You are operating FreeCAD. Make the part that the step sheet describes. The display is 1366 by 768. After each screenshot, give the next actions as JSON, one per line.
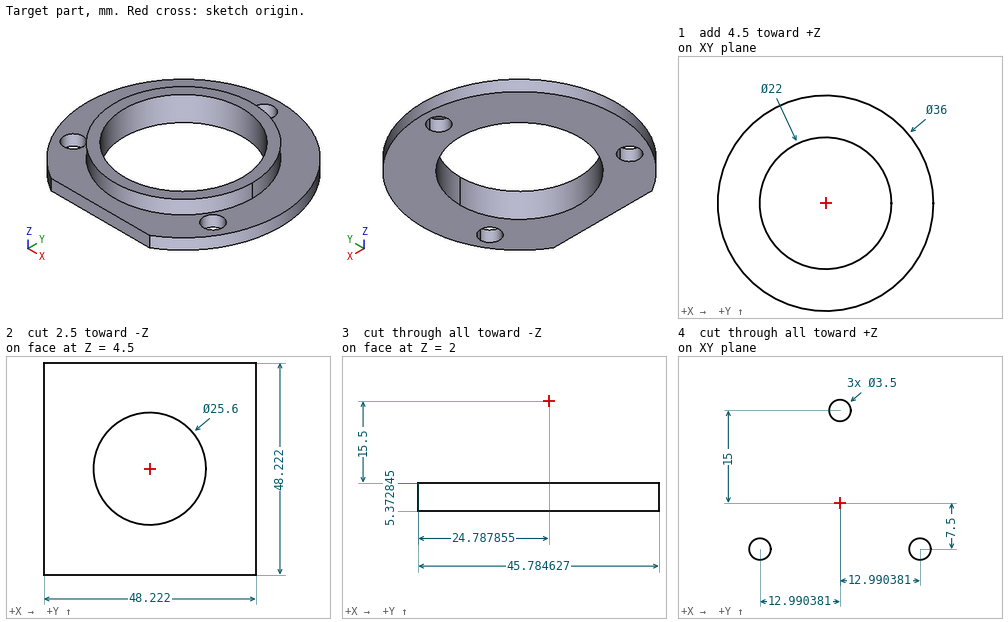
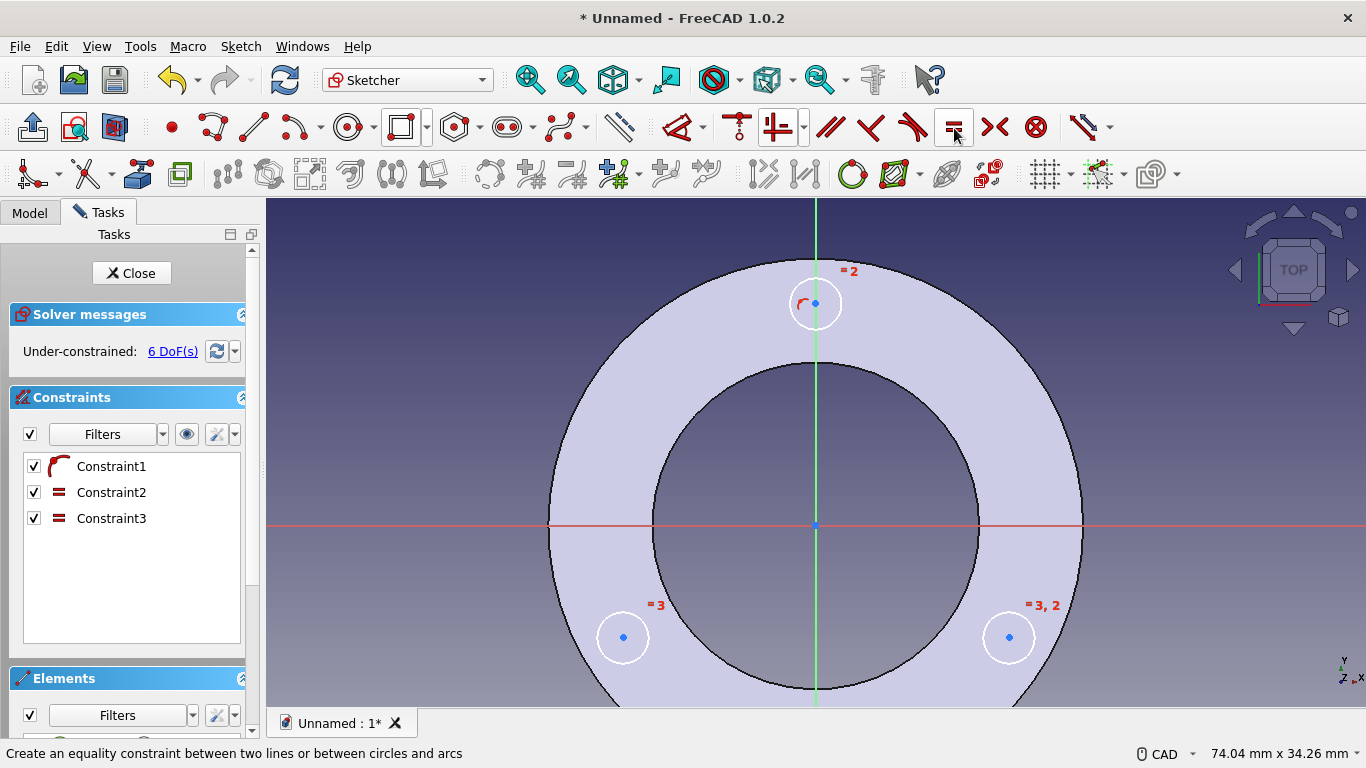
{"action": "left_click", "coordinate": [1009, 638]}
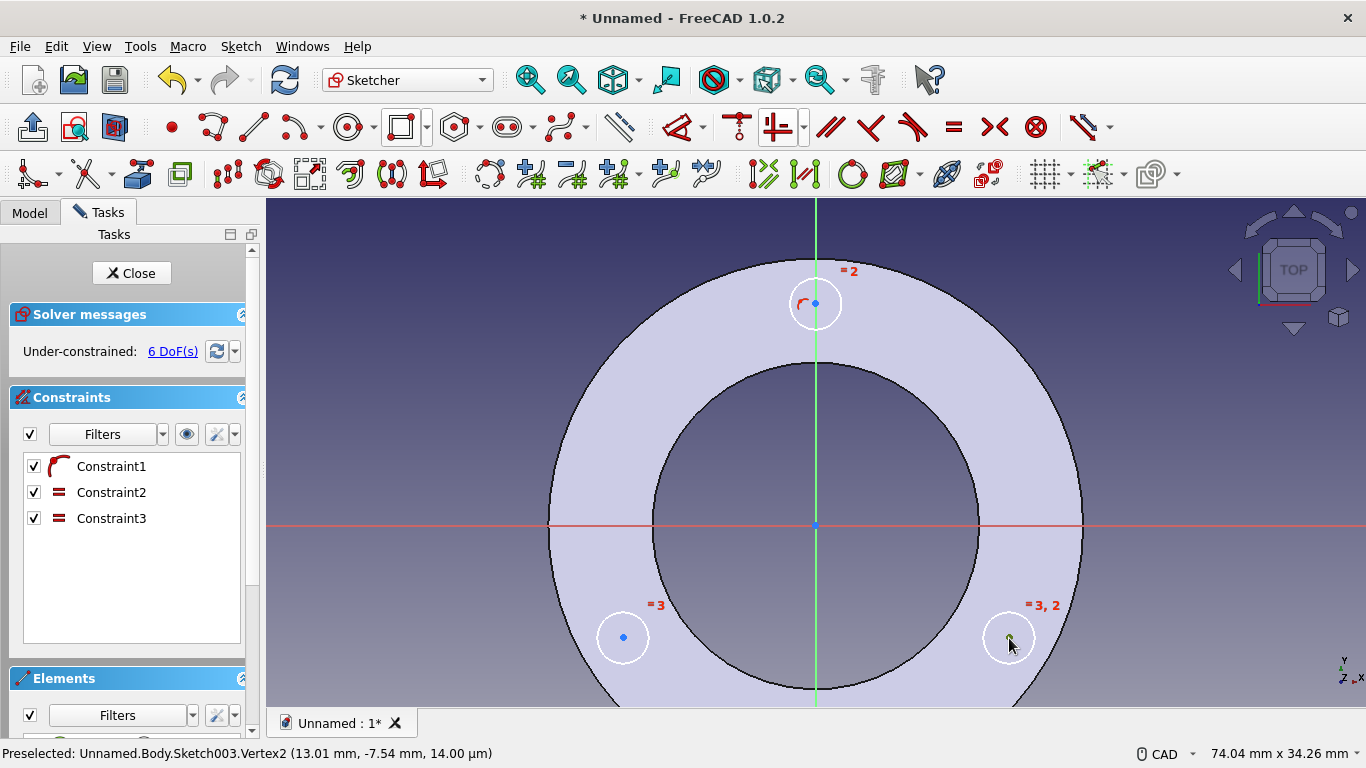
{"action": "left_click", "coordinate": [623, 638]}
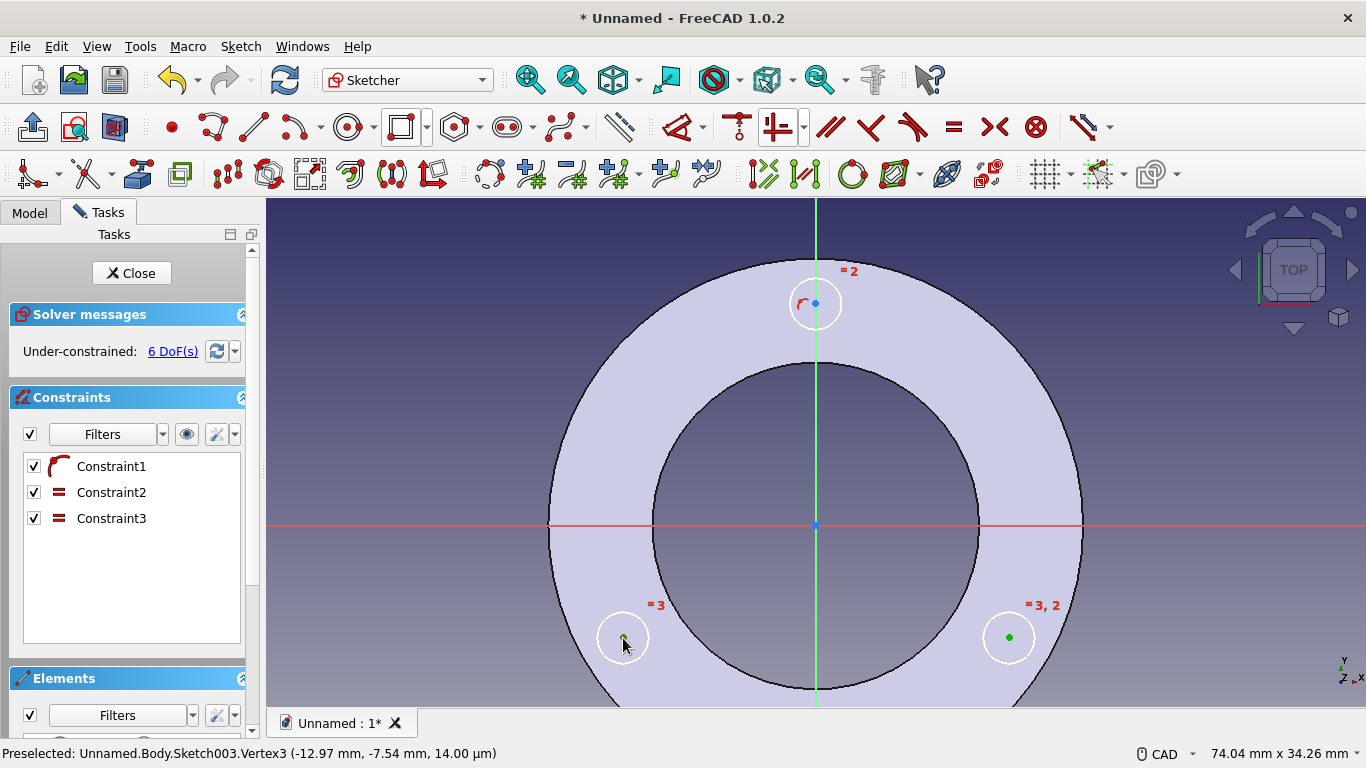
{"action": "left_click", "coordinate": [804, 128]}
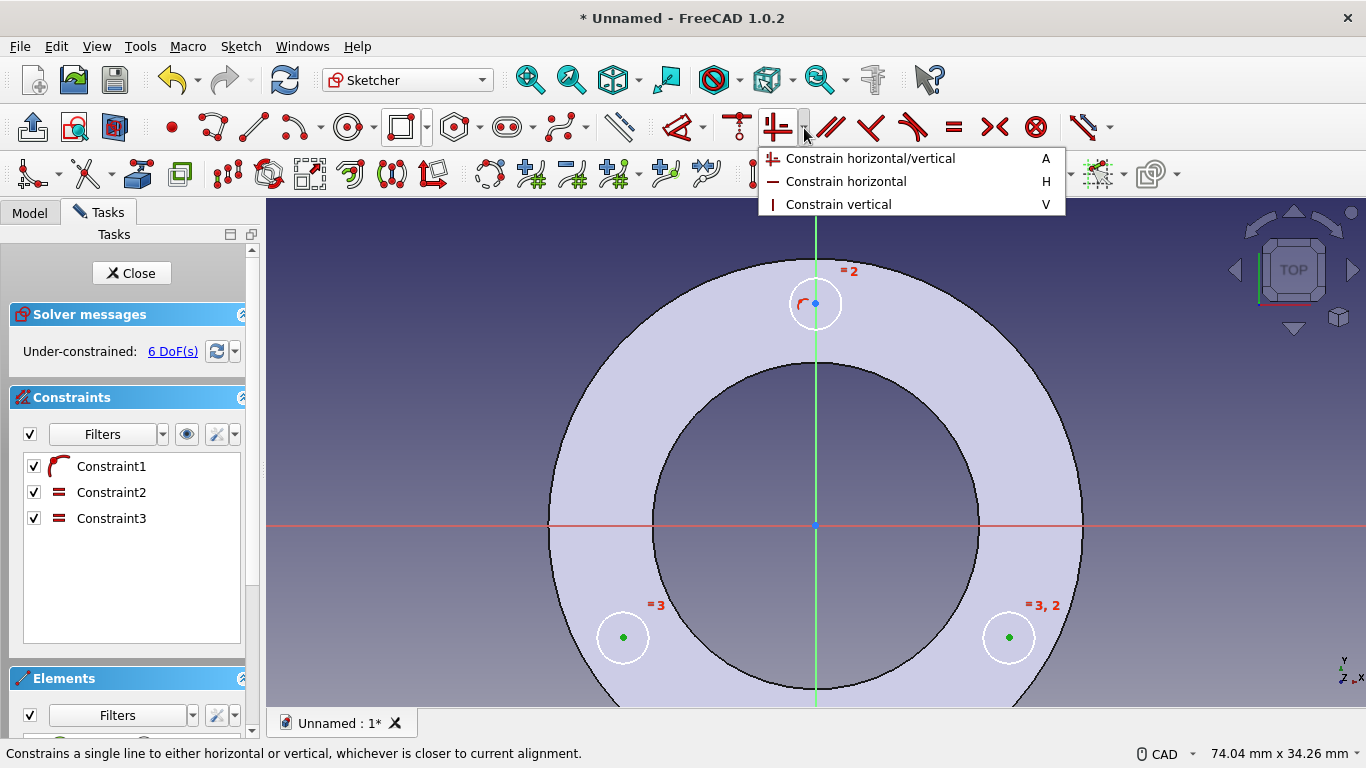
{"action": "left_click", "coordinate": [912, 182]}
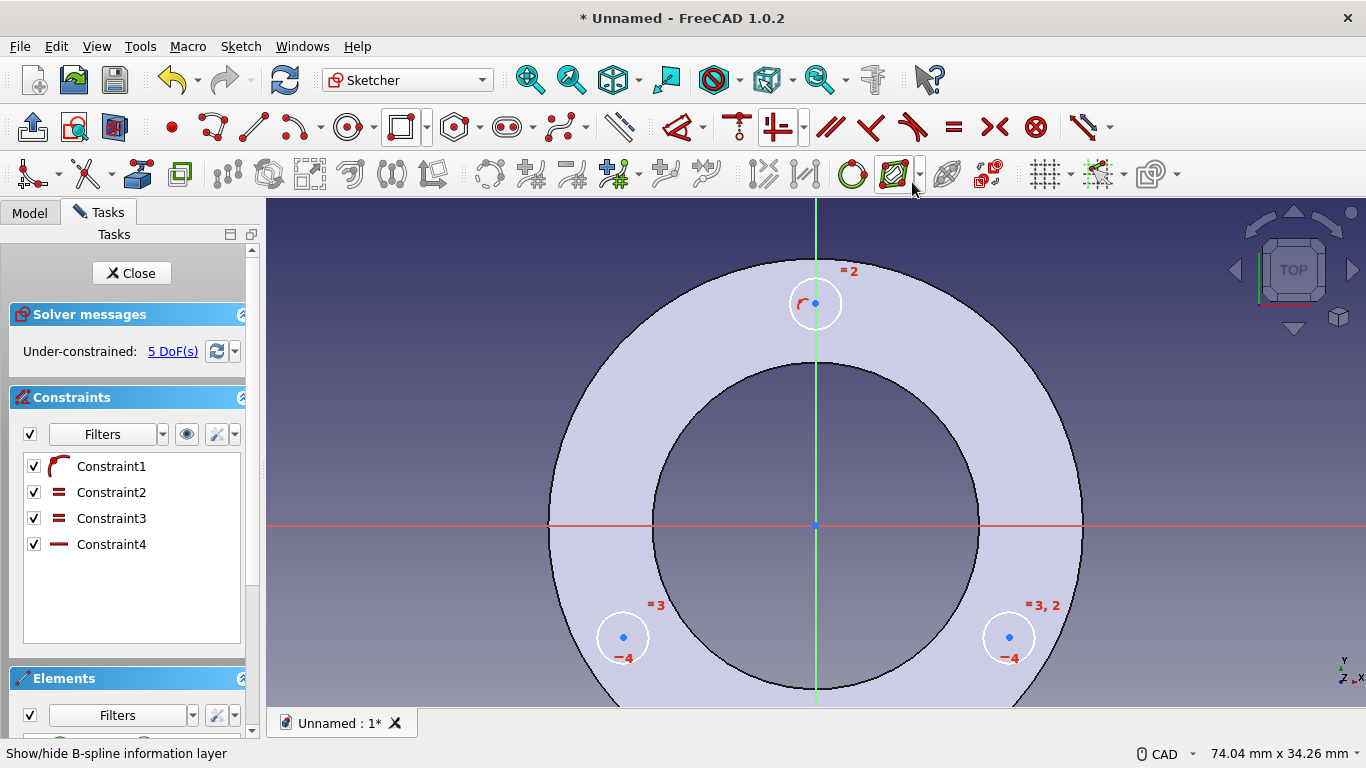
{"action": "left_click", "coordinate": [676, 128]}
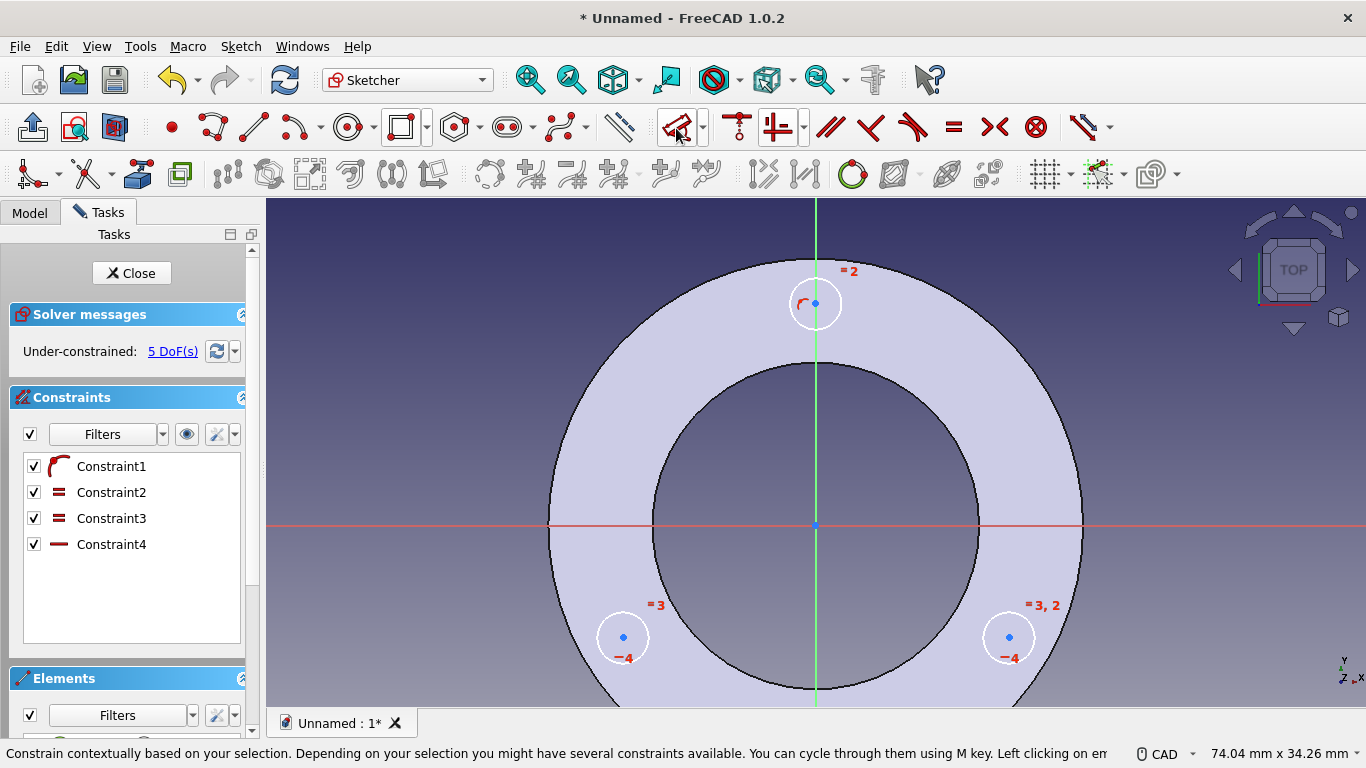
{"action": "left_click", "coordinate": [834, 286]}
{"action": "left_click", "coordinate": [857, 264]}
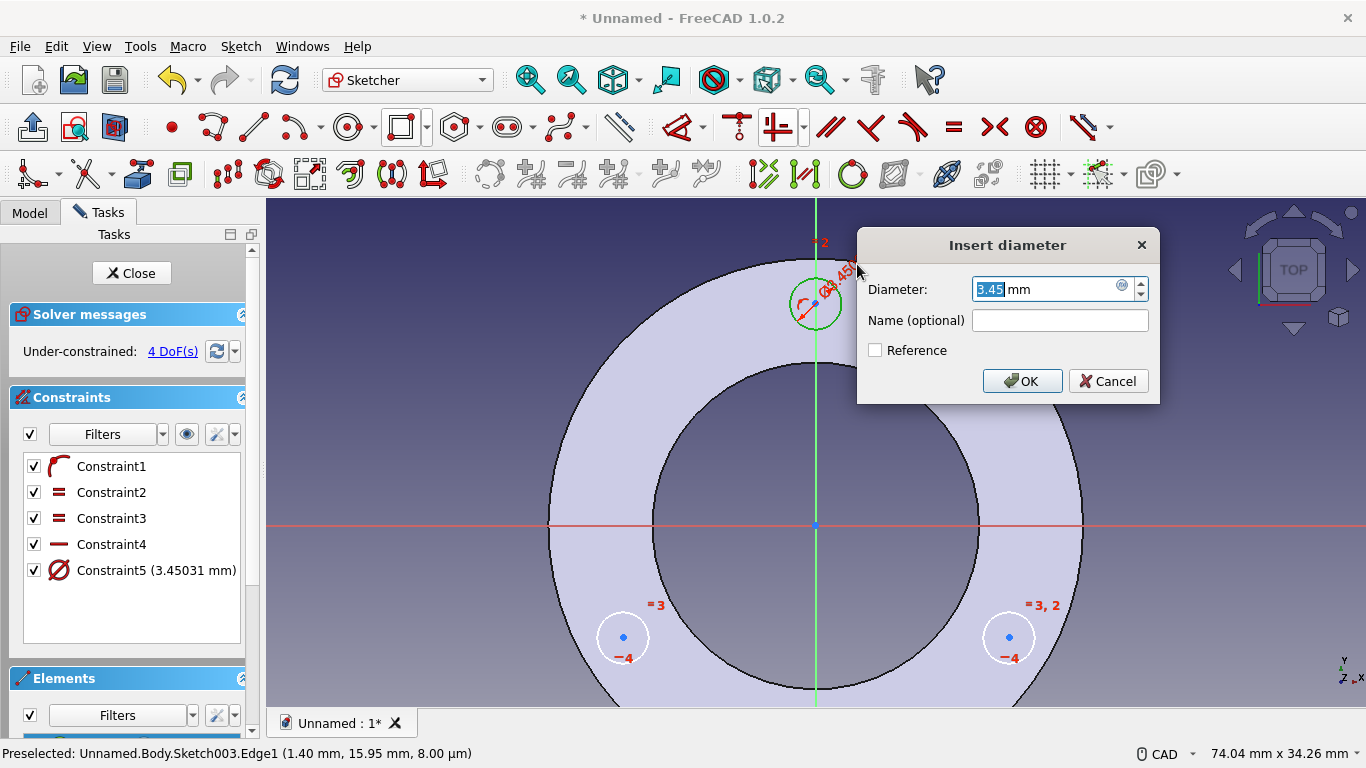
{"action": "type", "text": "3.5"}
{"action": "key", "text": "Return"}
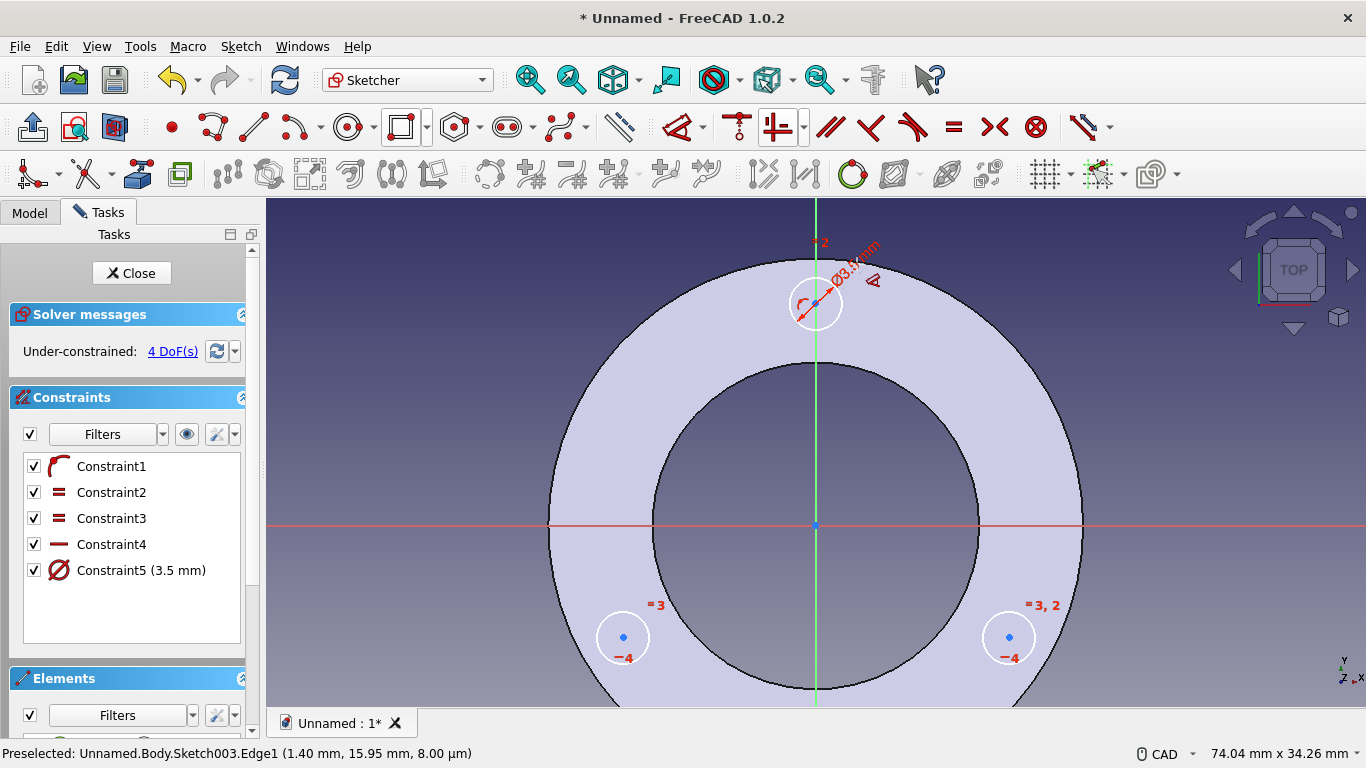
{"action": "left_click", "coordinate": [816, 304]}
{"action": "left_click", "coordinate": [850, 415]}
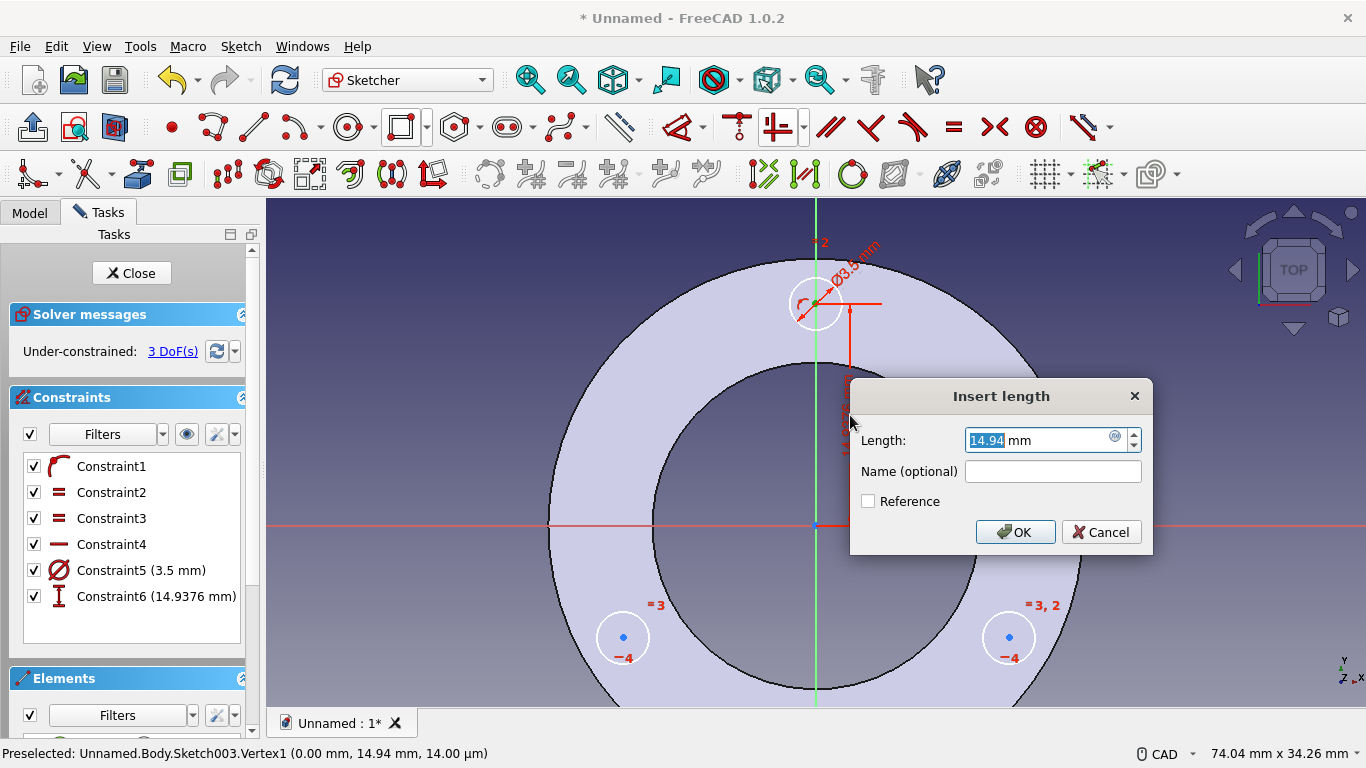
{"action": "type", "text": "15"}
{"action": "key", "text": "Return"}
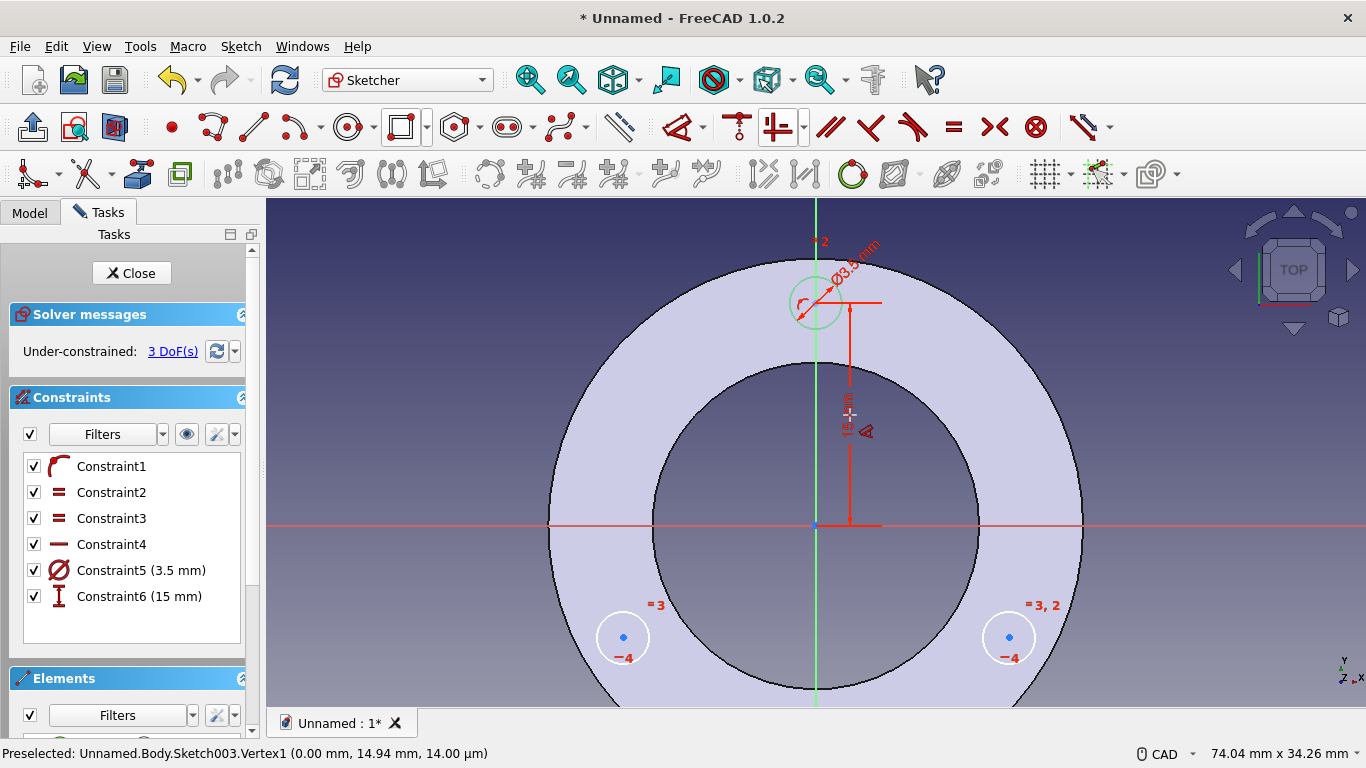
{"action": "left_click", "coordinate": [1009, 638]}
{"action": "left_click", "coordinate": [1043, 582]}